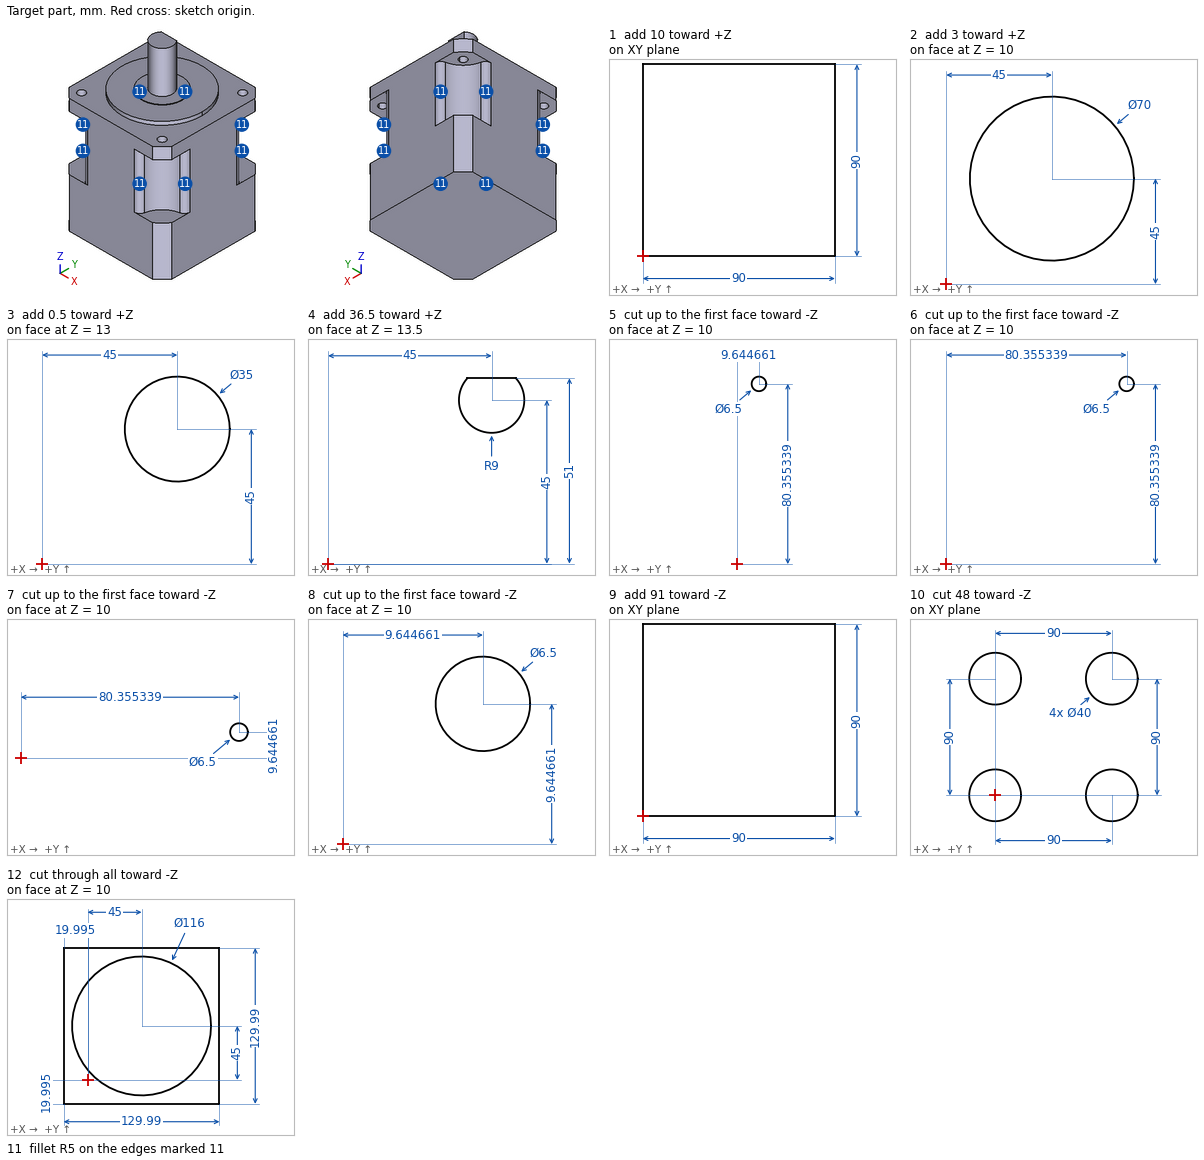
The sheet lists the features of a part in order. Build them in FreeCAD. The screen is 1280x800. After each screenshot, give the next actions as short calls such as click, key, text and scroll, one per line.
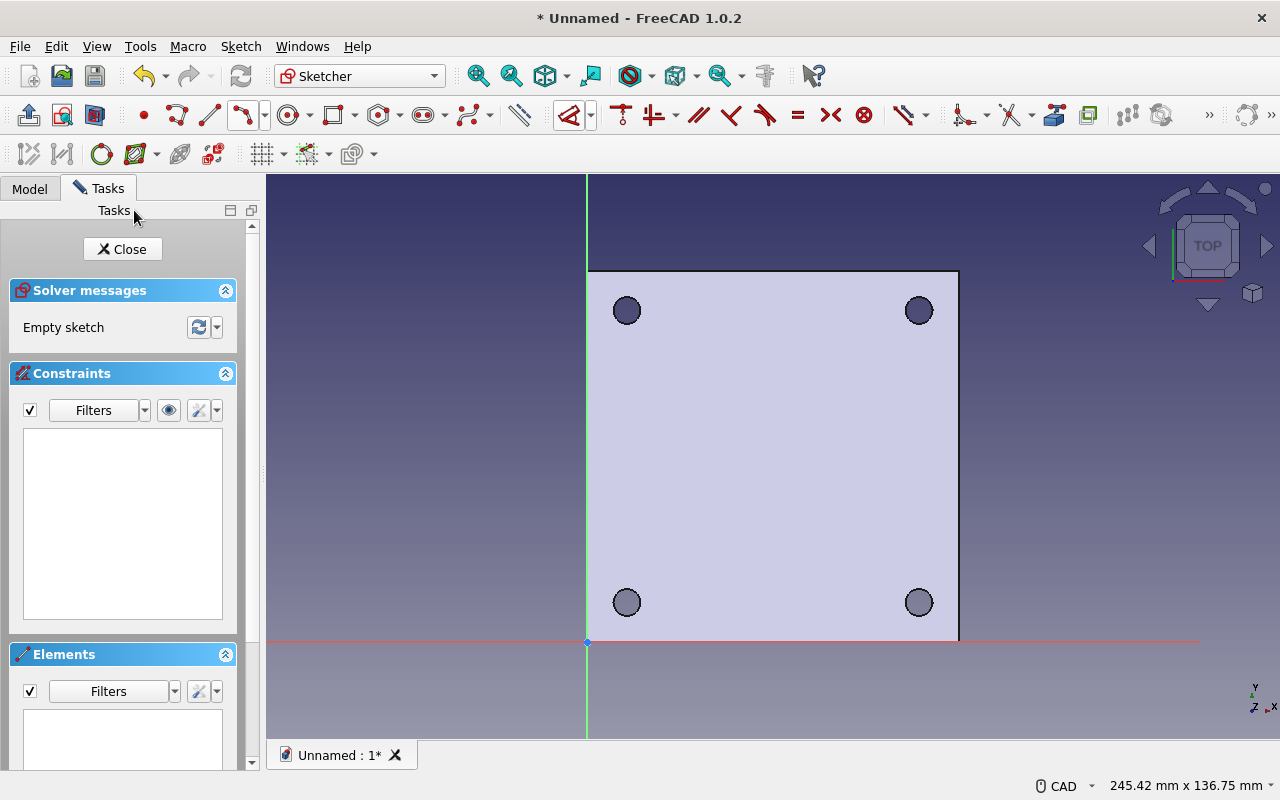
key(g)
key(r)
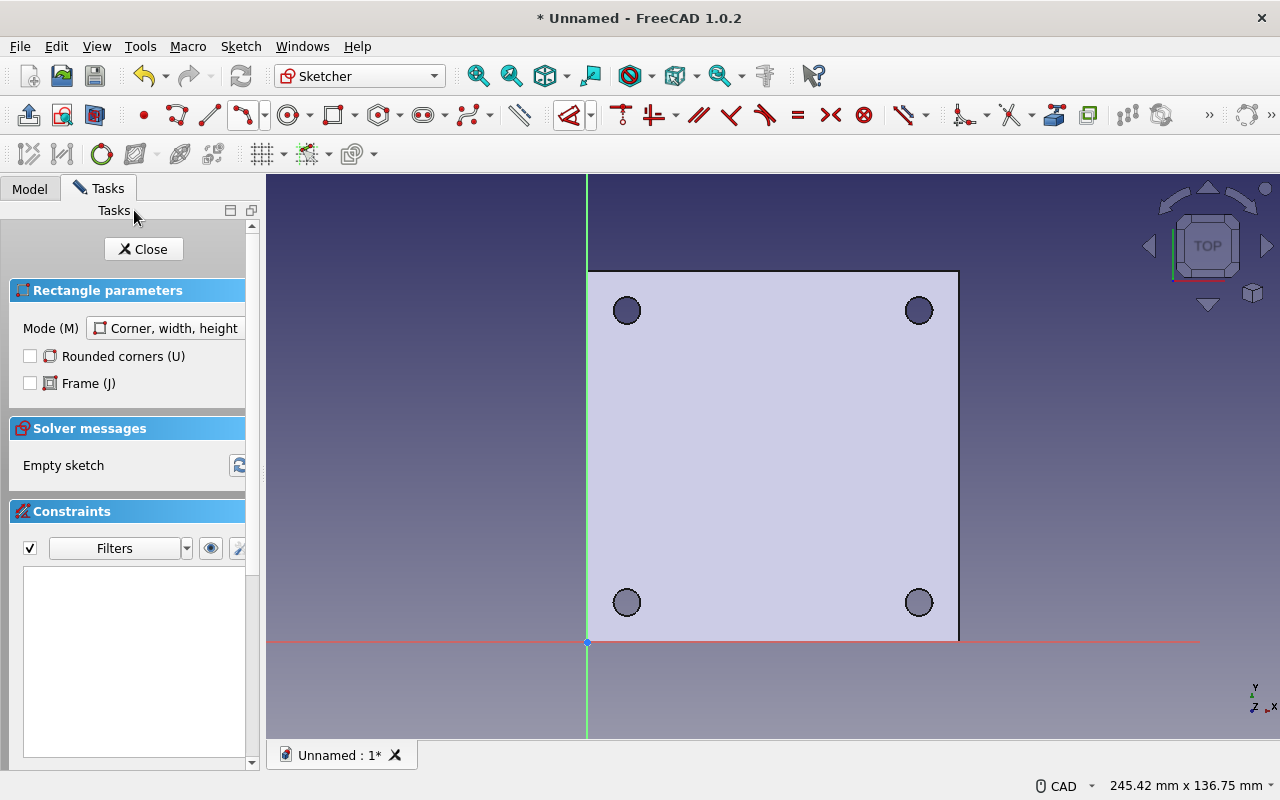
click(587, 642)
move(959, 271)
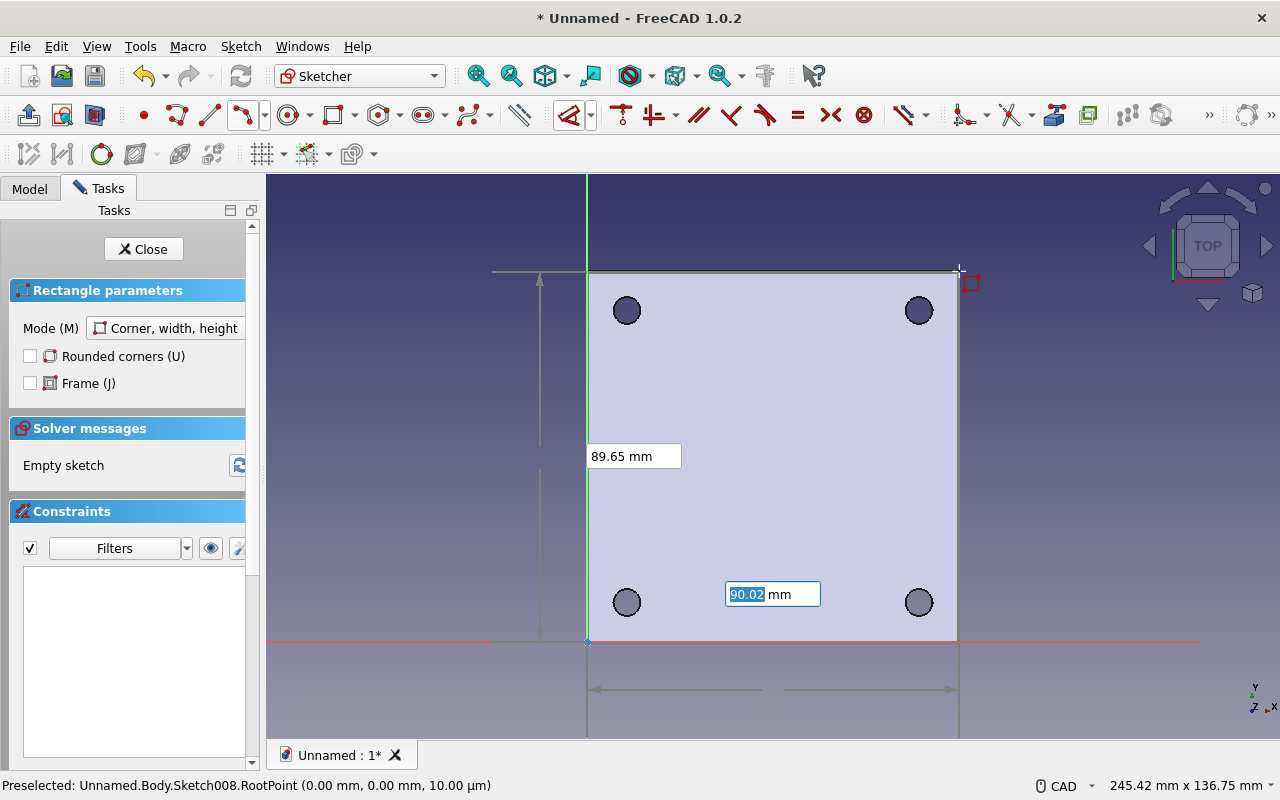
text(90)
key(Tab)
text(90)
key(Return)
key(Escape)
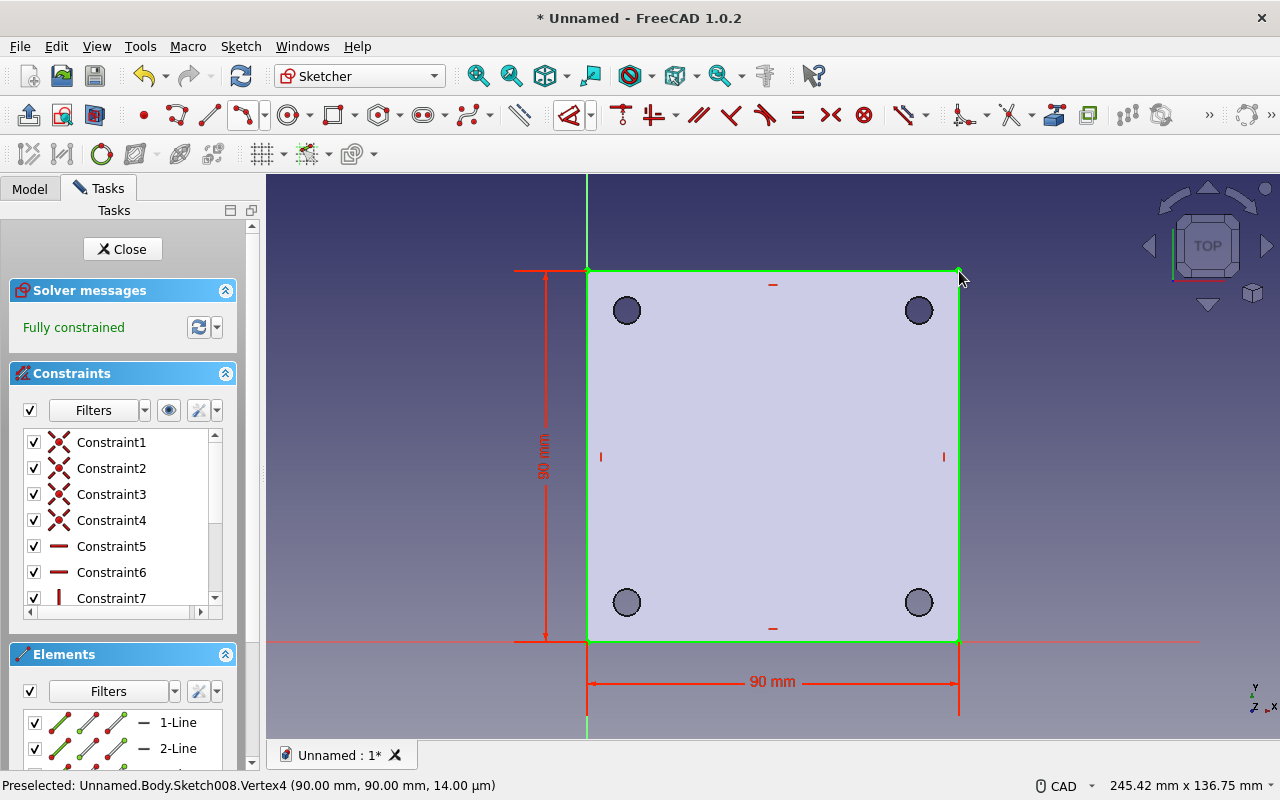
click(123, 249)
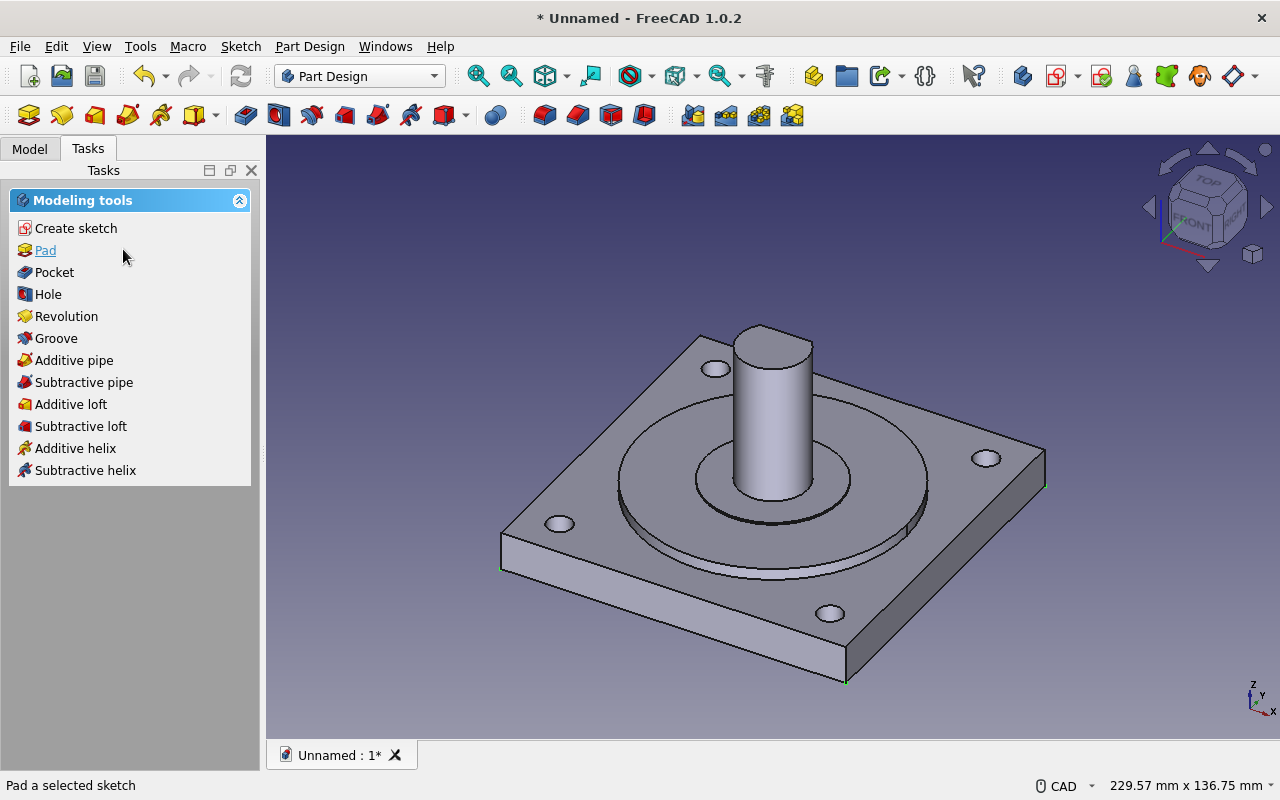
click(29, 116)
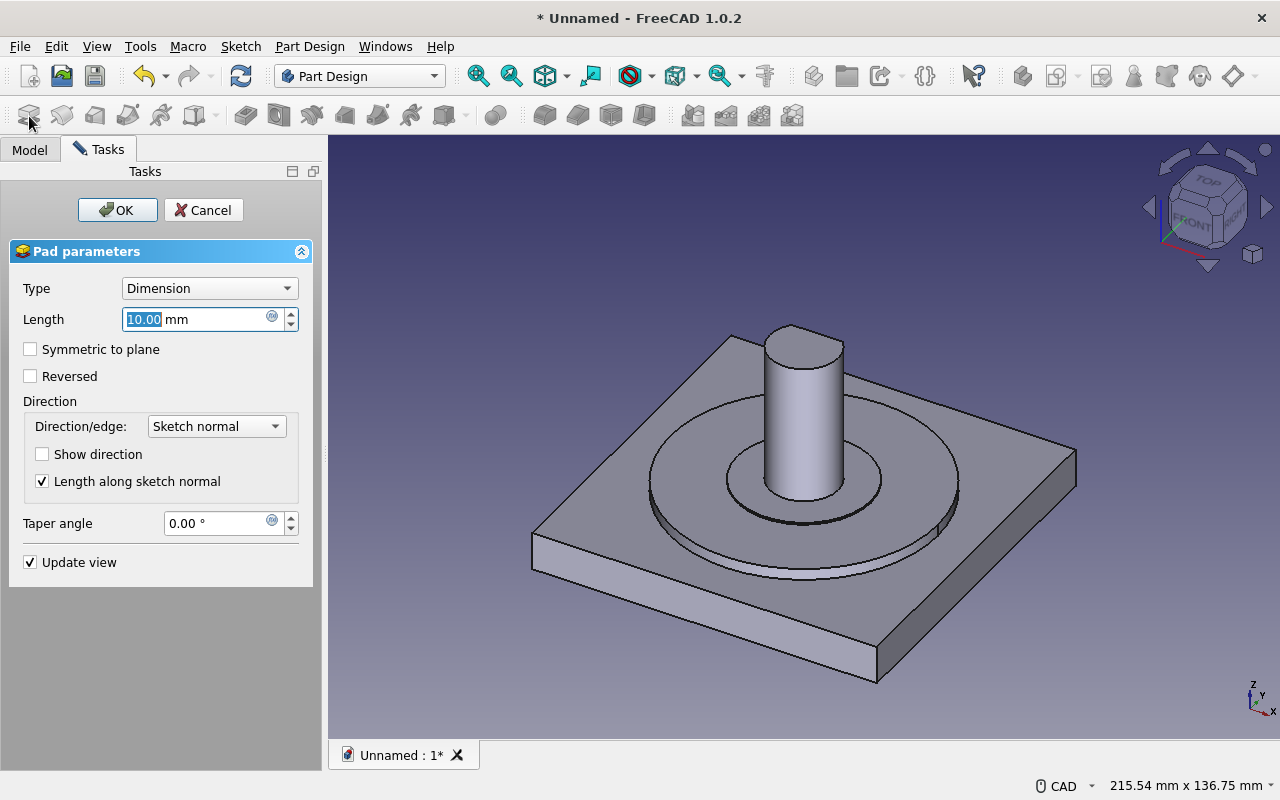
text(91)
key(Tab)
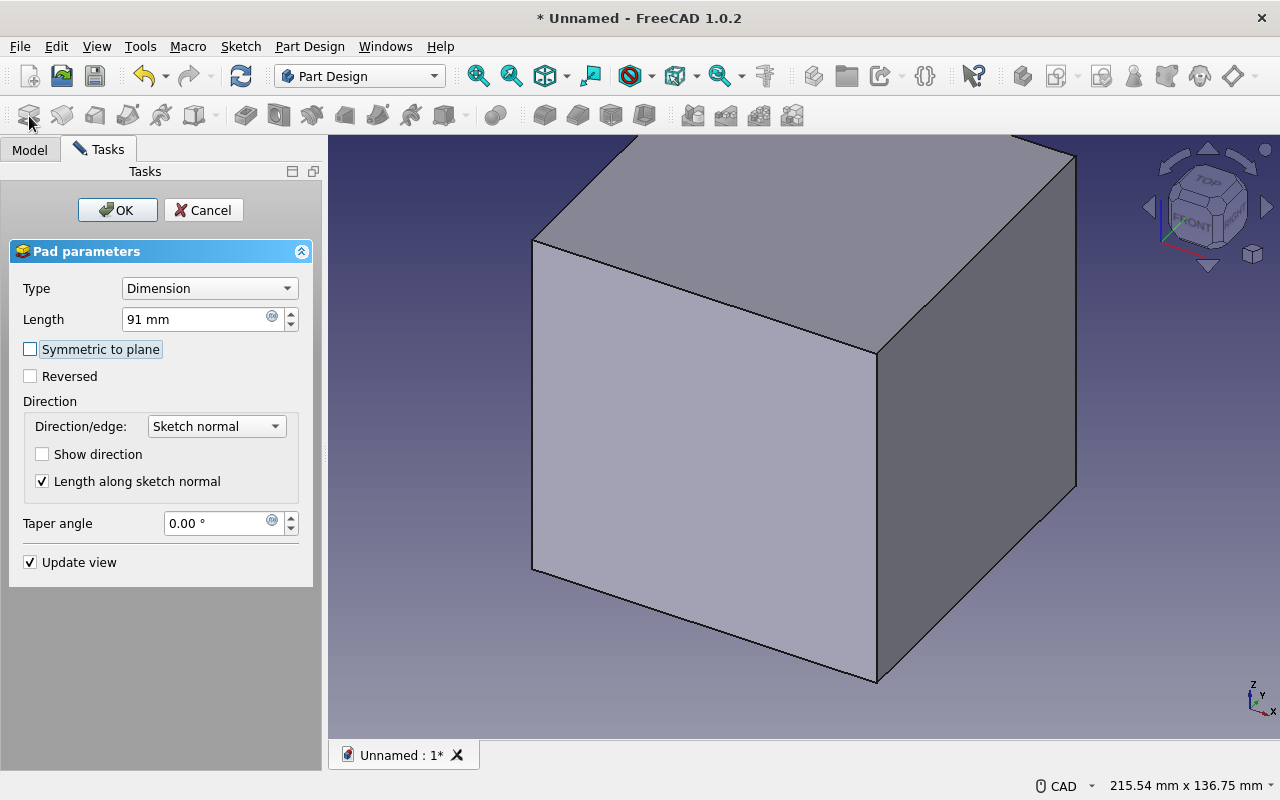
click(31, 376)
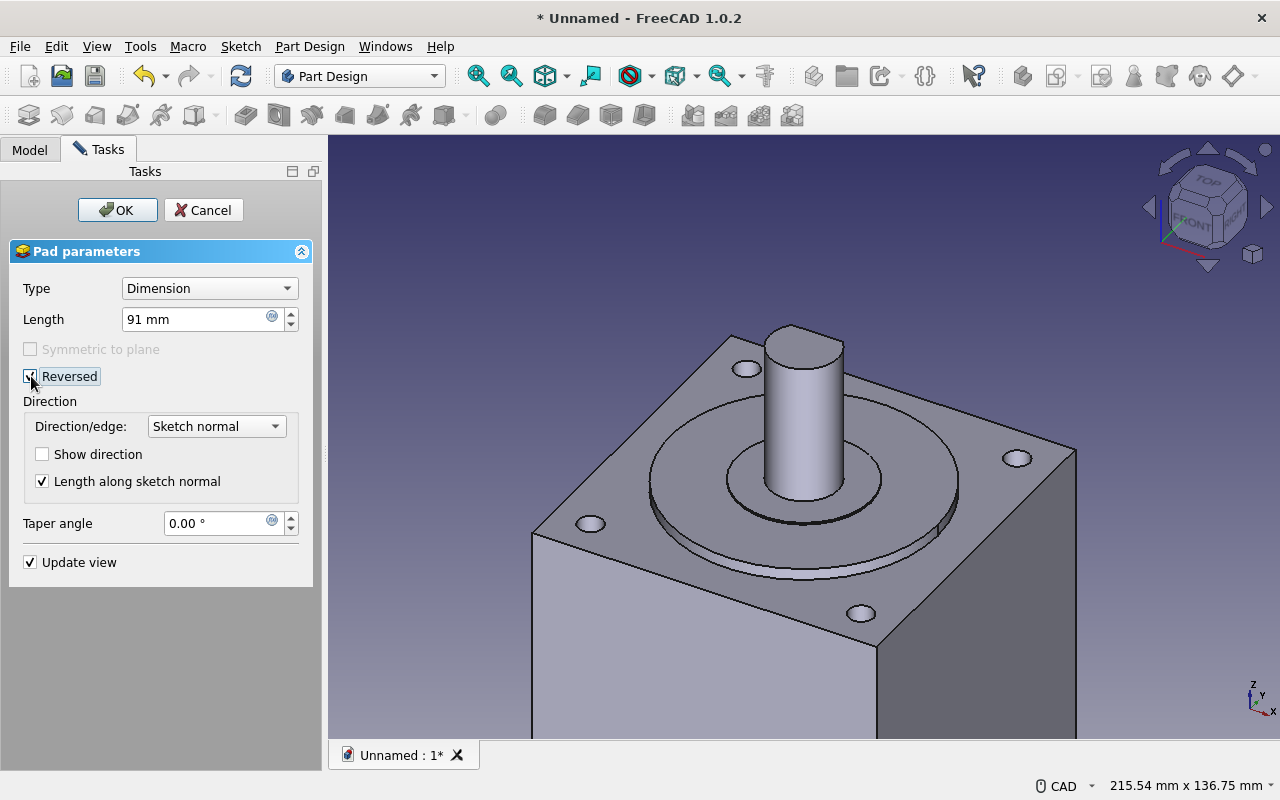
click(118, 210)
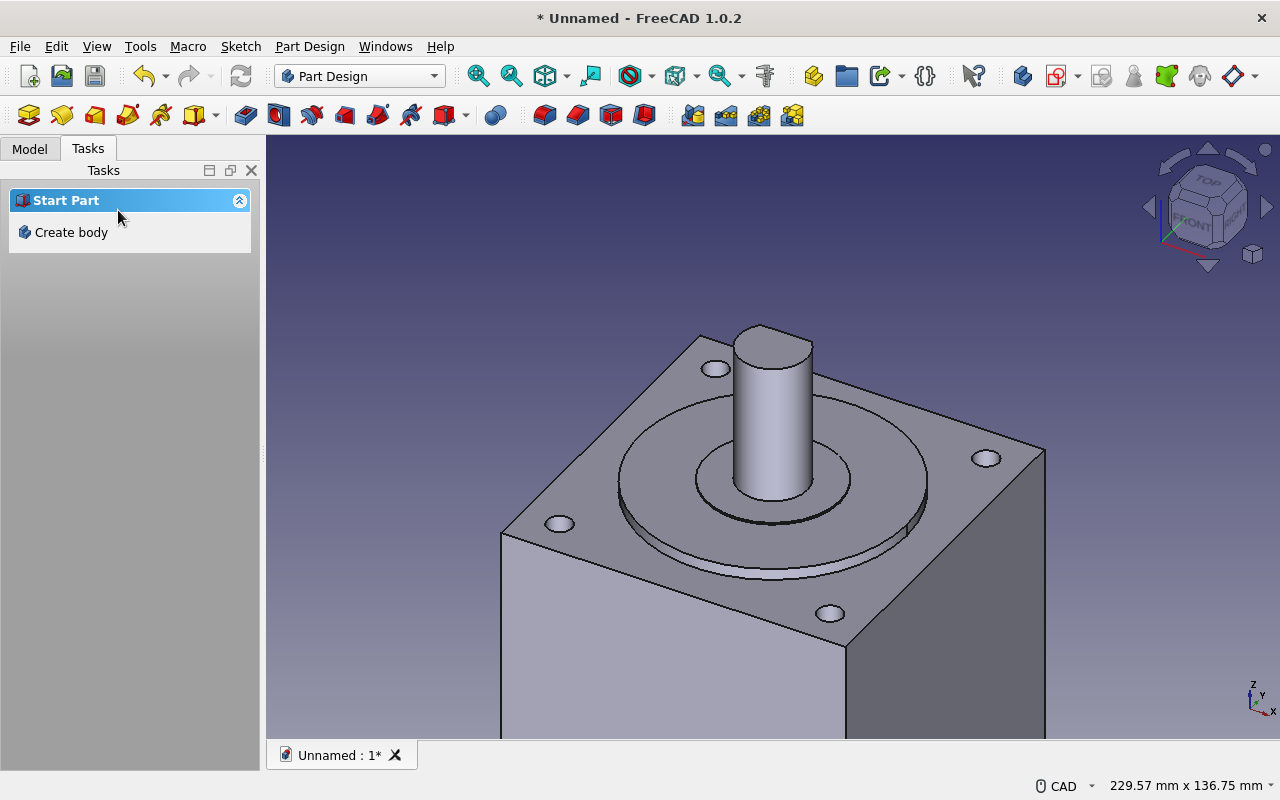
key(v)
key(f)